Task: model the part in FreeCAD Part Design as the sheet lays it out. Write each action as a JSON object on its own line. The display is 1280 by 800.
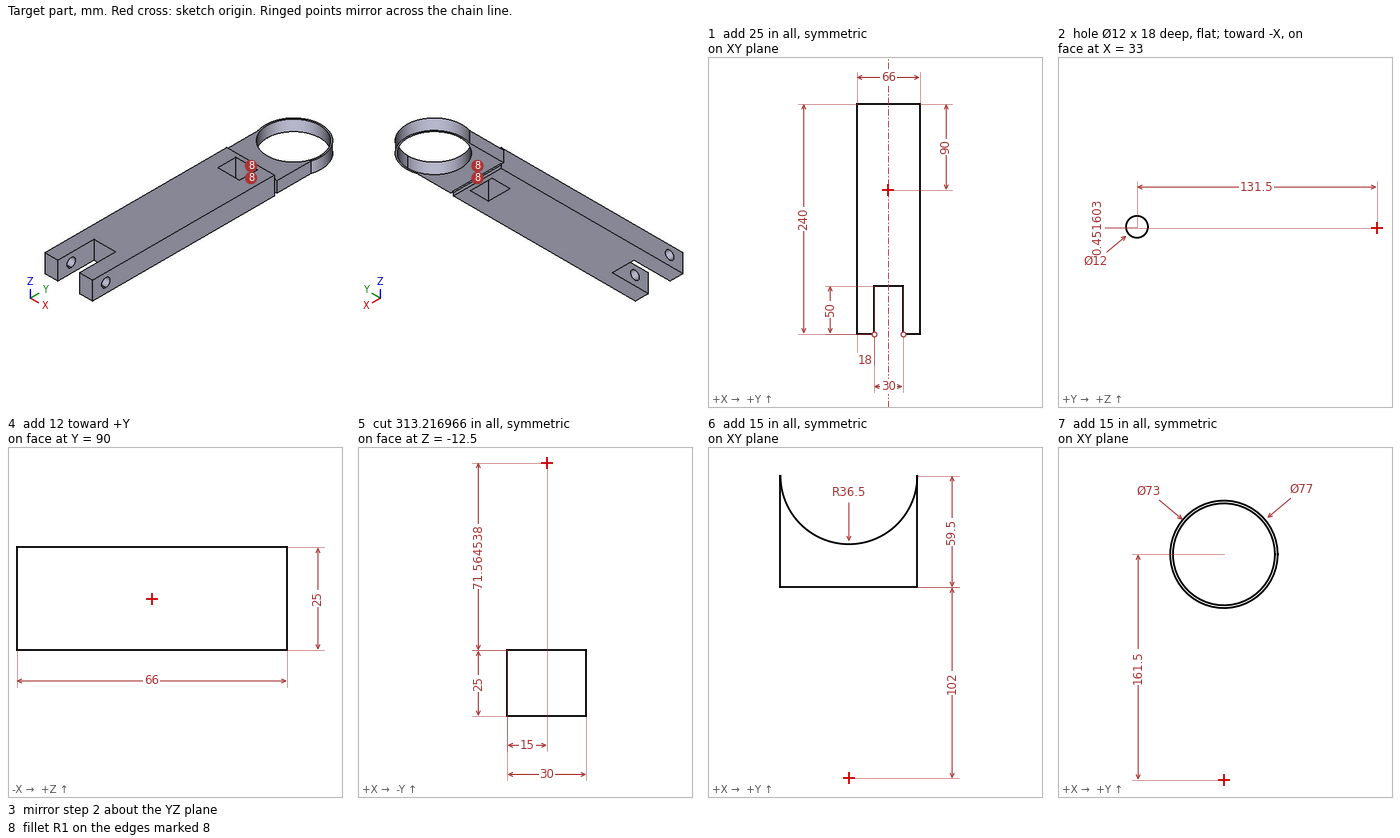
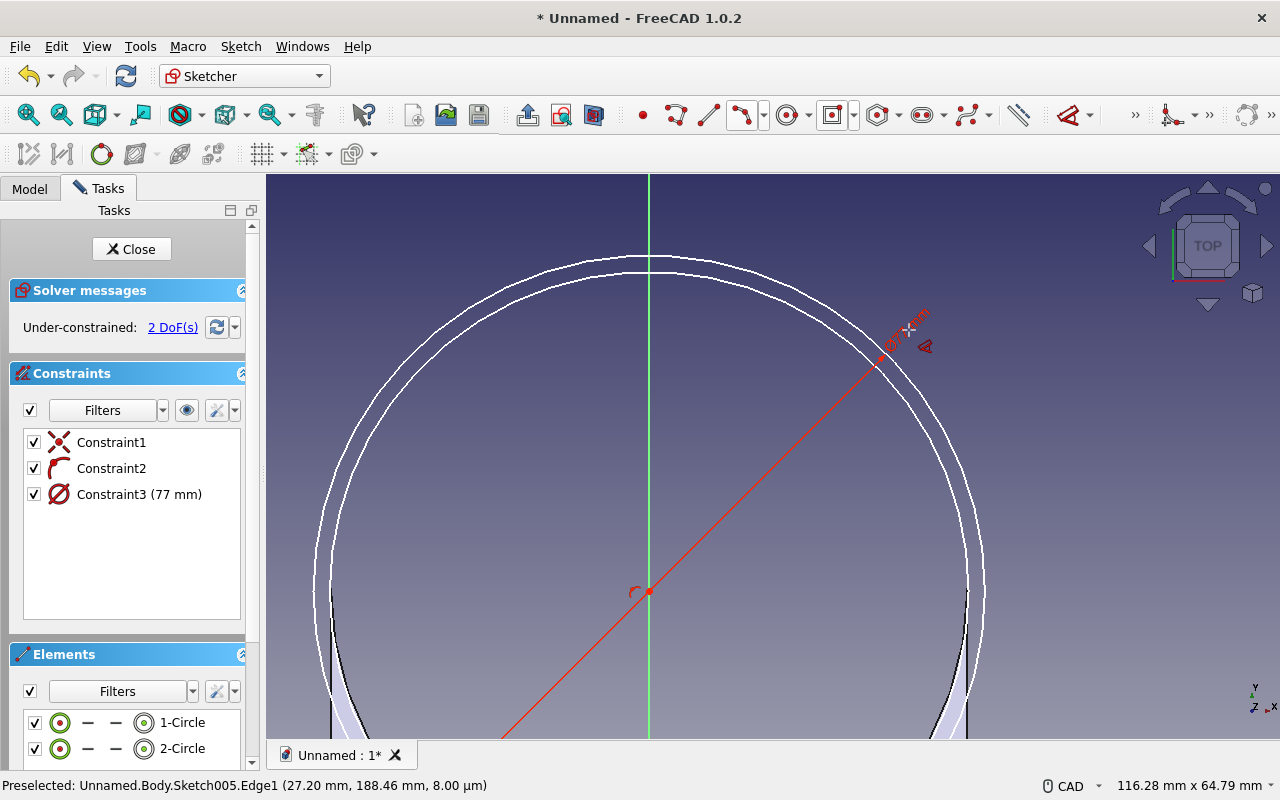
{"action": "left_click", "coordinate": [874, 365]}
{"action": "left_click", "coordinate": [986, 491]}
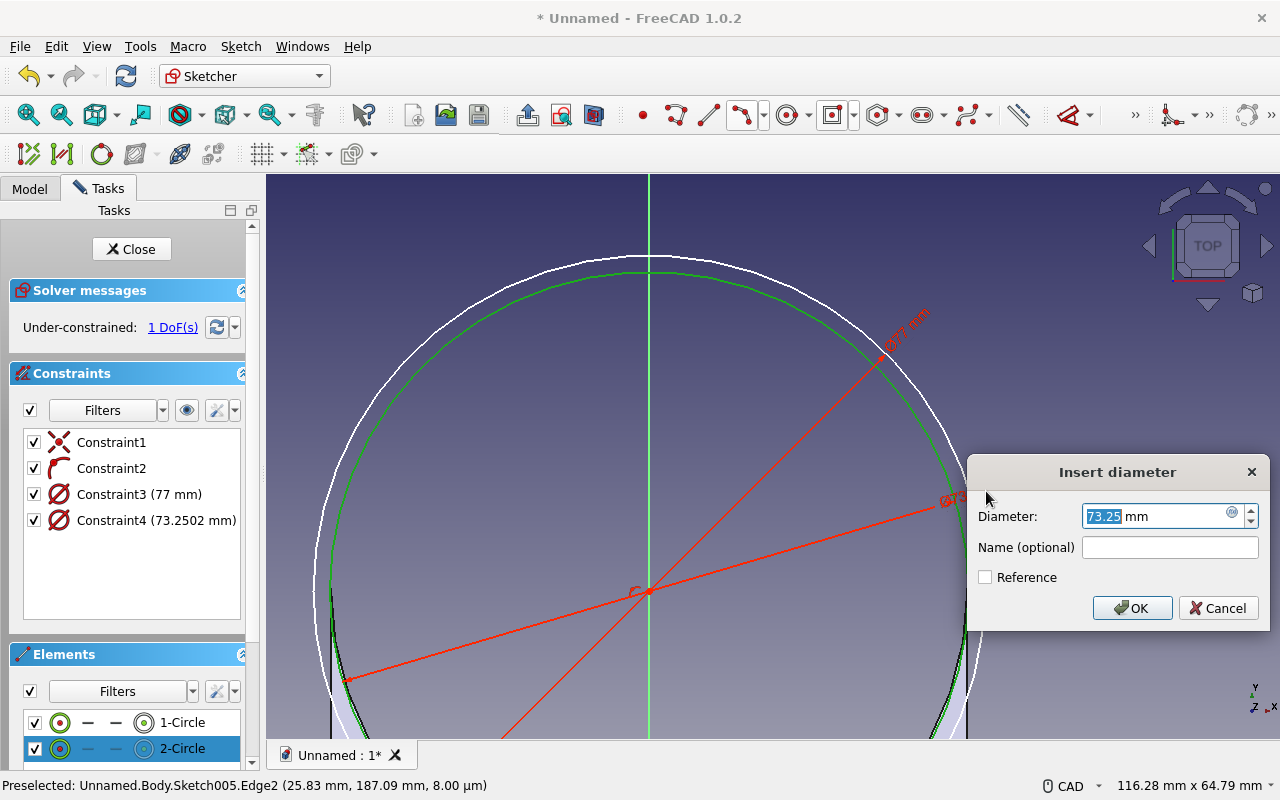
{"action": "type", "text": "73"}
{"action": "key", "text": "Return"}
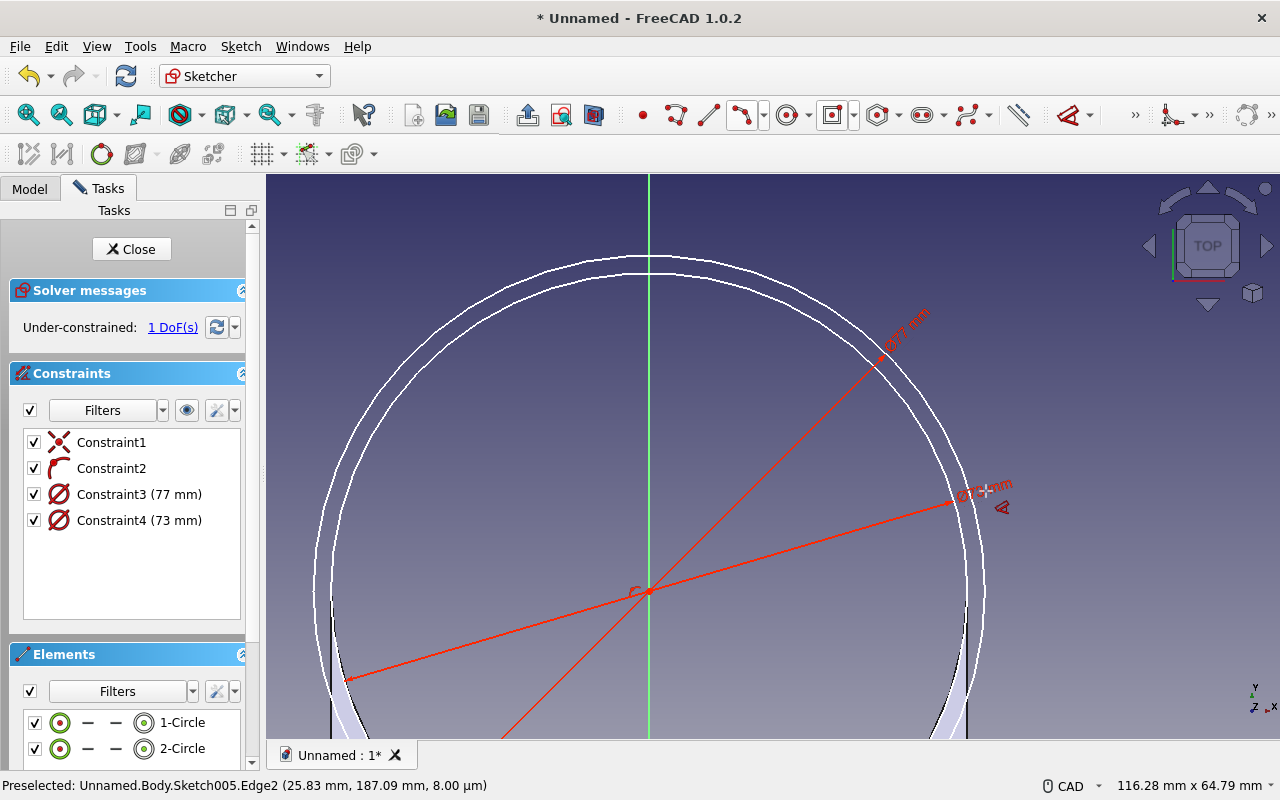
{"action": "left_click", "coordinate": [649, 591]}
{"action": "left_click", "coordinate": [683, 651]}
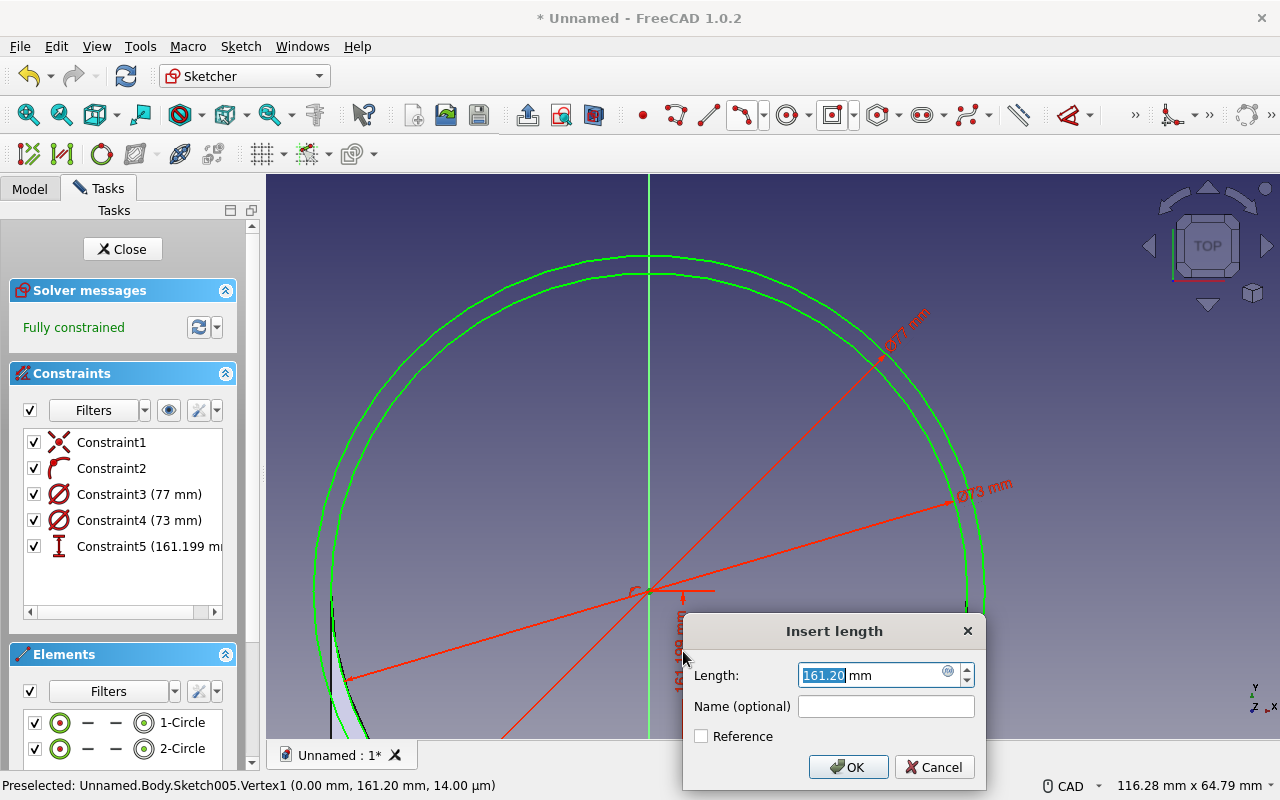
{"action": "type", "text": "161.5"}
{"action": "key", "text": "Return"}
{"action": "key", "text": "Escape"}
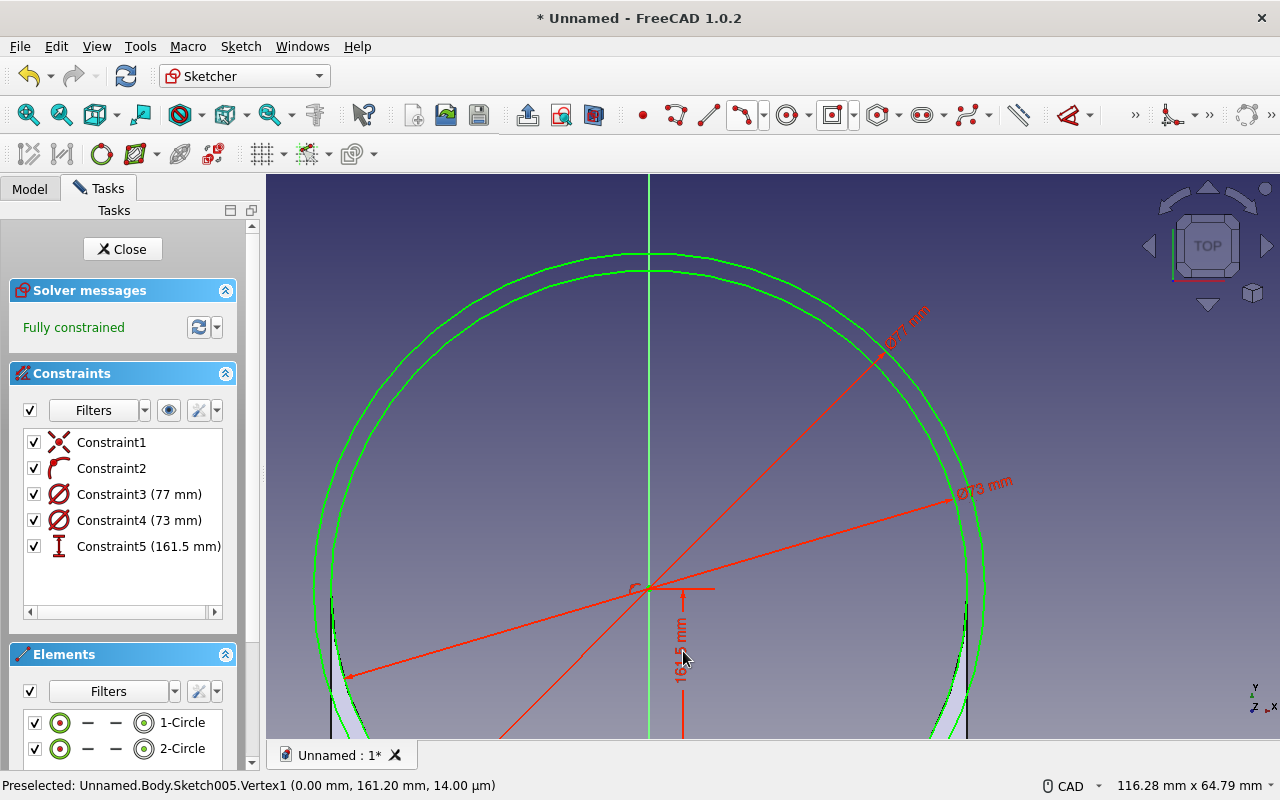
{"action": "left_click", "coordinate": [123, 249]}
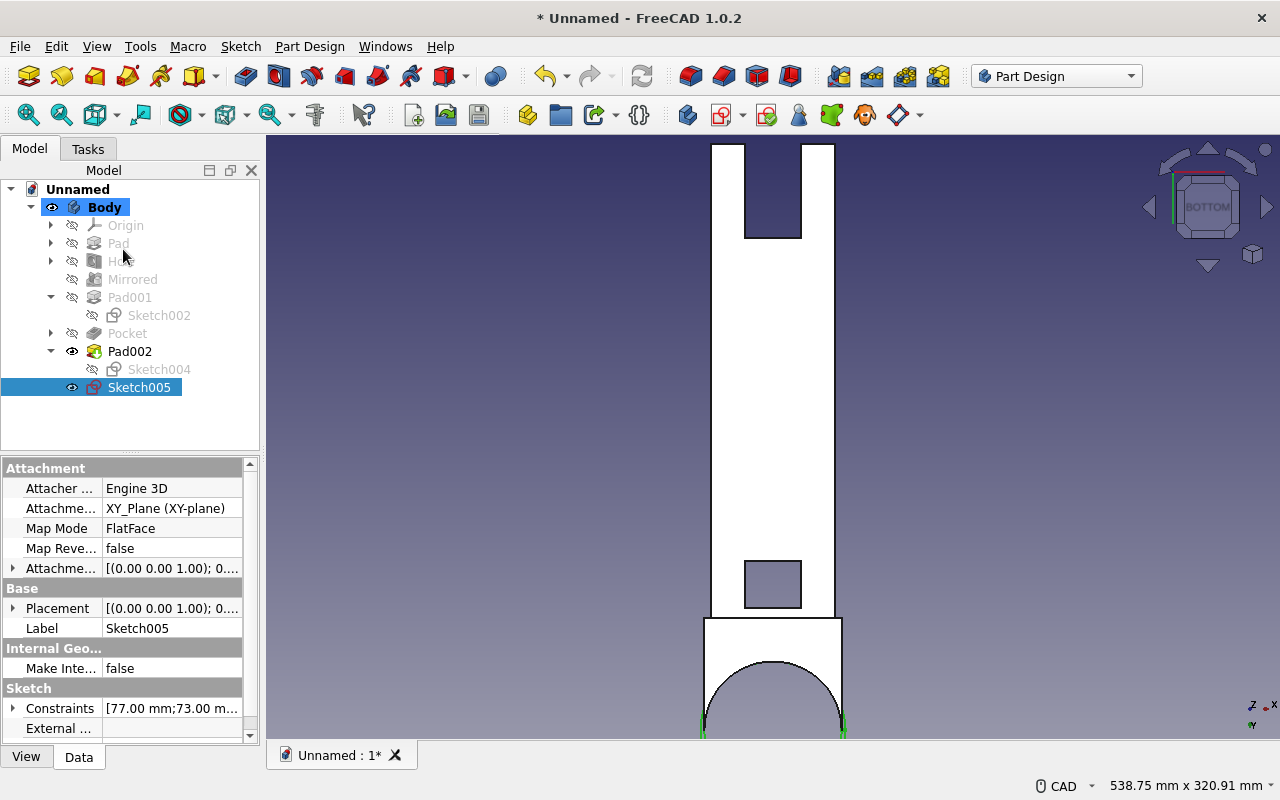
{"action": "left_click", "coordinate": [29, 76]}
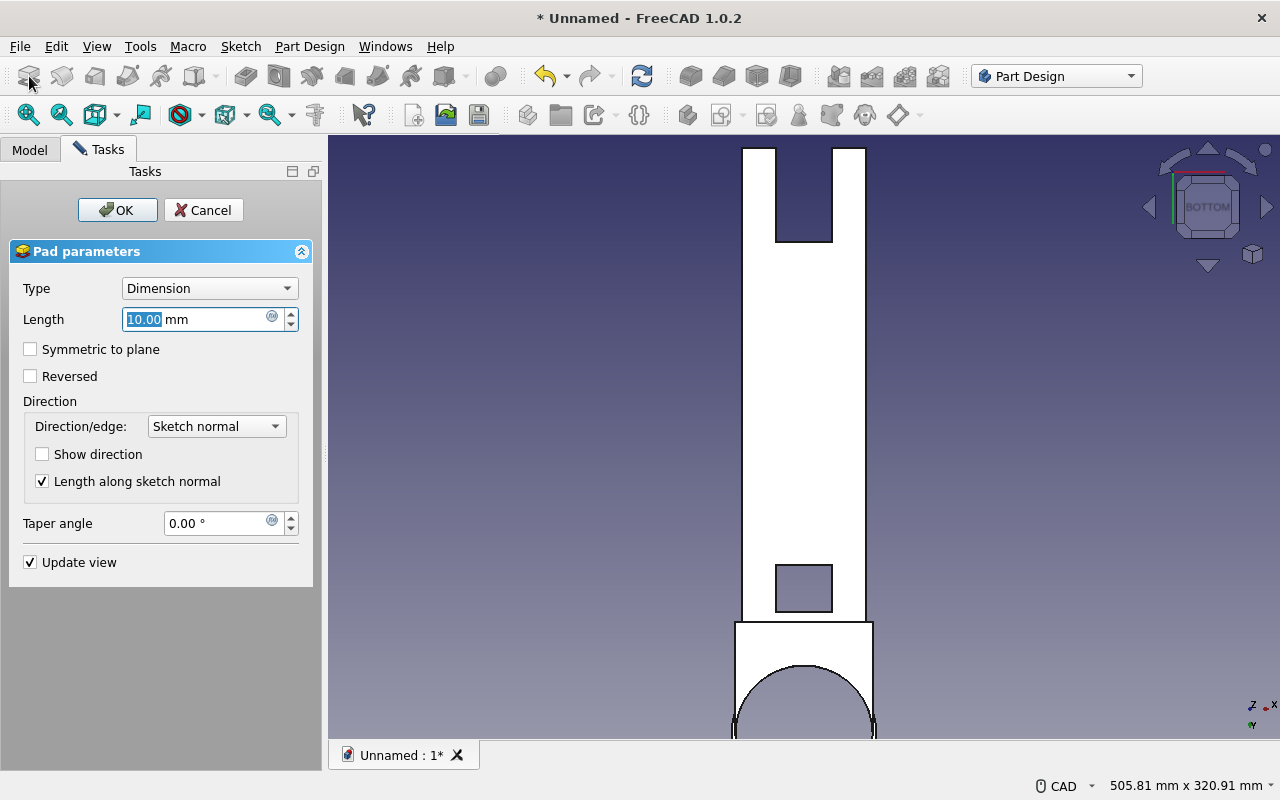
{"action": "type", "text": "15"}
{"action": "key", "text": "Tab"}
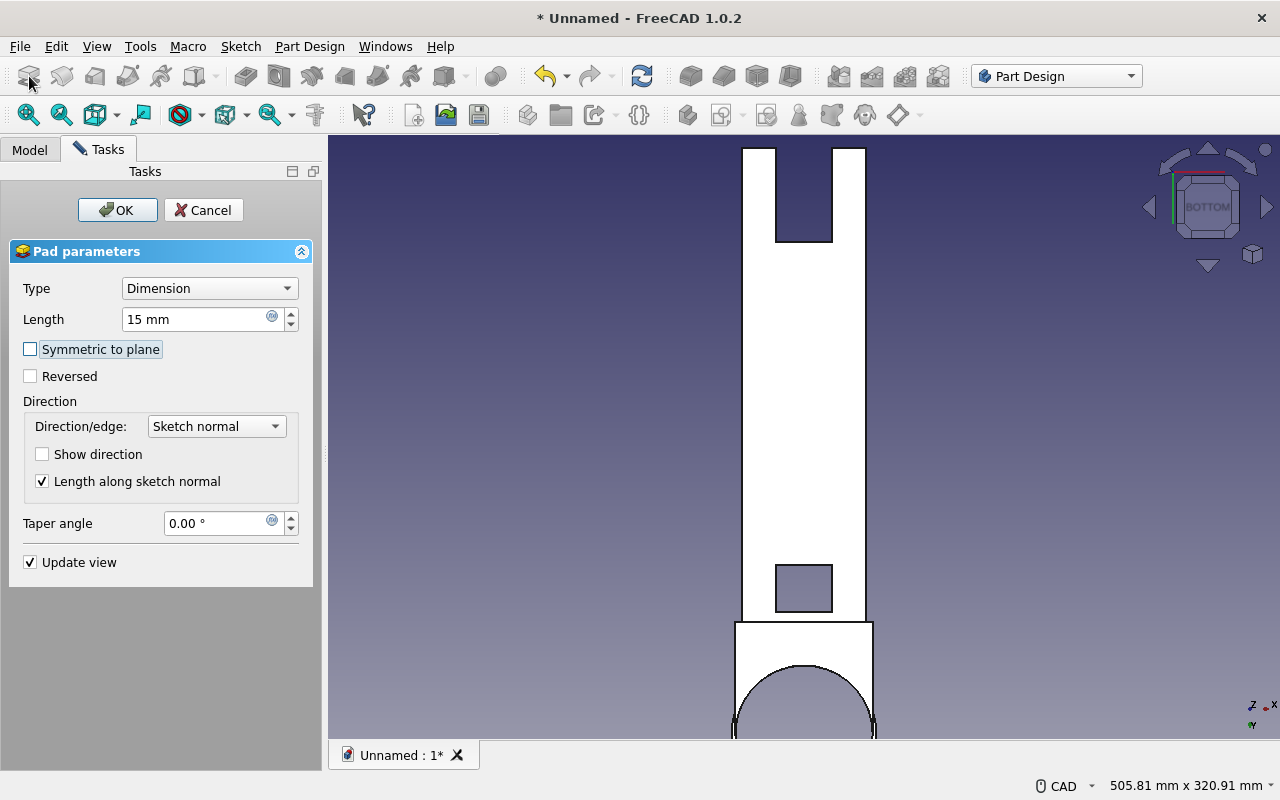
{"action": "left_click", "coordinate": [31, 349]}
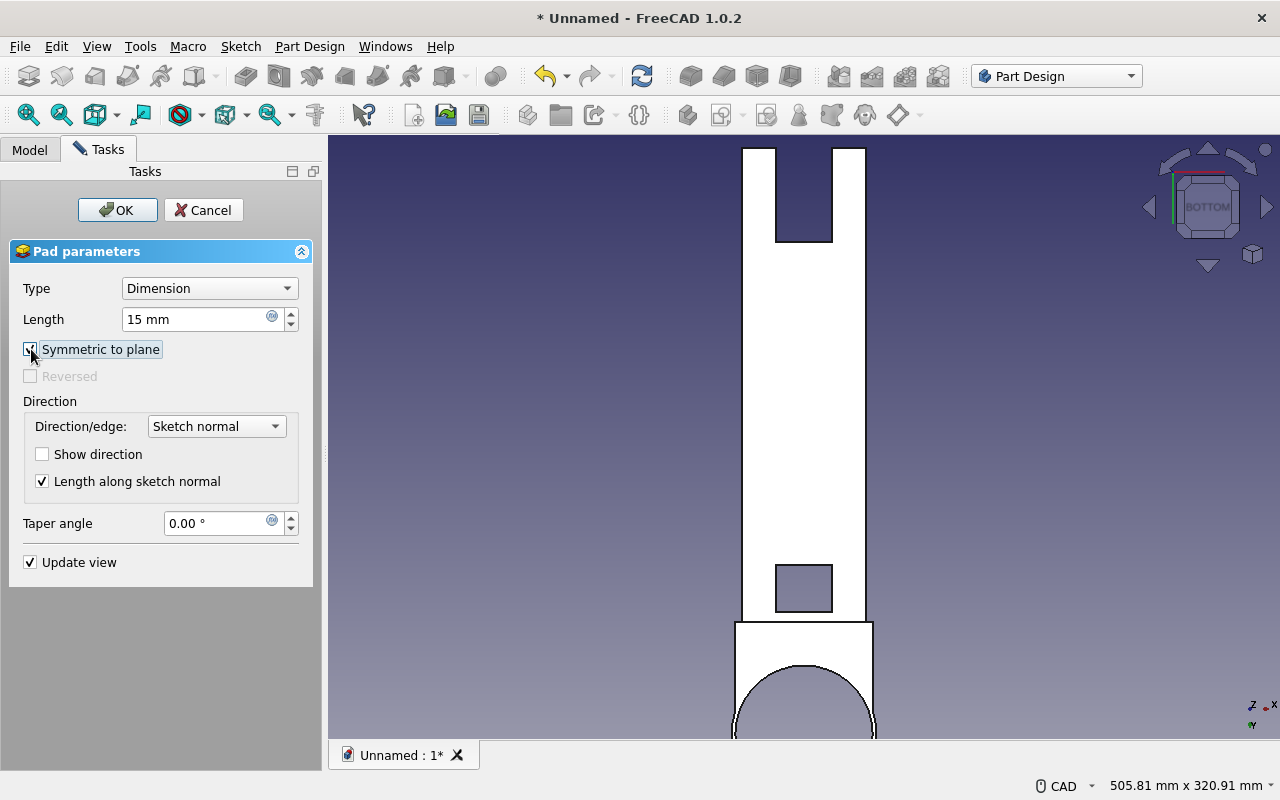
{"action": "left_click", "coordinate": [118, 210]}